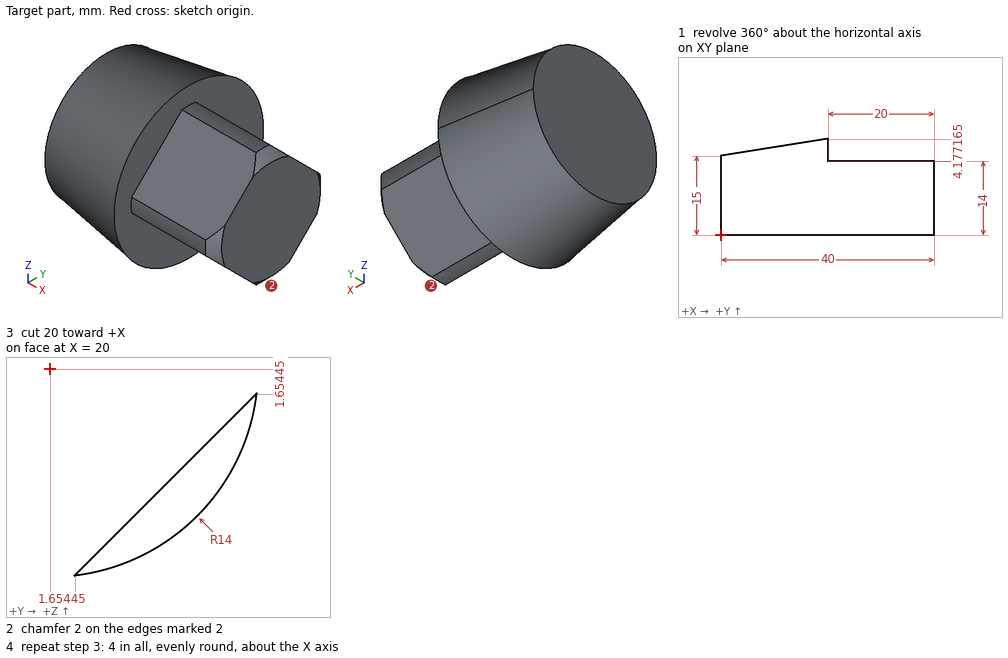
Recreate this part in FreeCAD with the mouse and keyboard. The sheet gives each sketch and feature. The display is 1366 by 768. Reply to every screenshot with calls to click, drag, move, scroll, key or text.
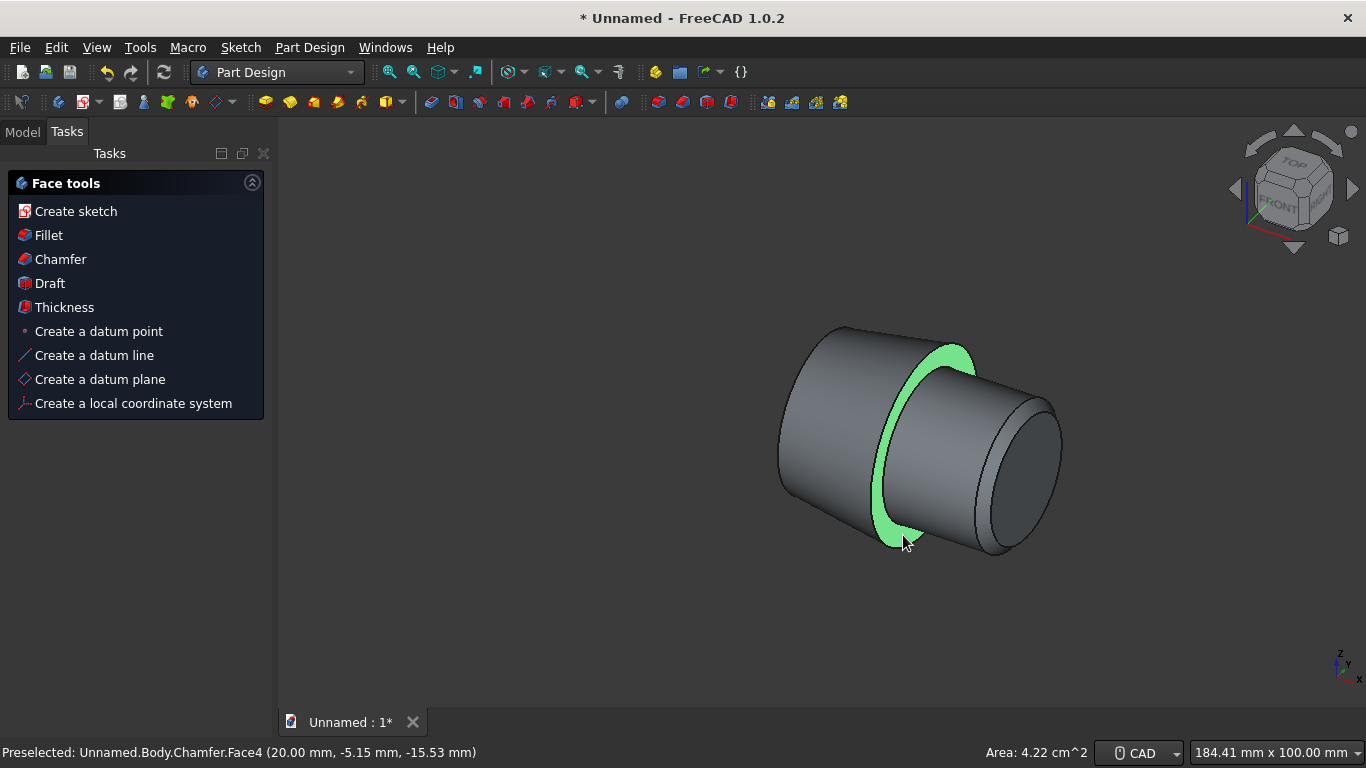
click(84, 102)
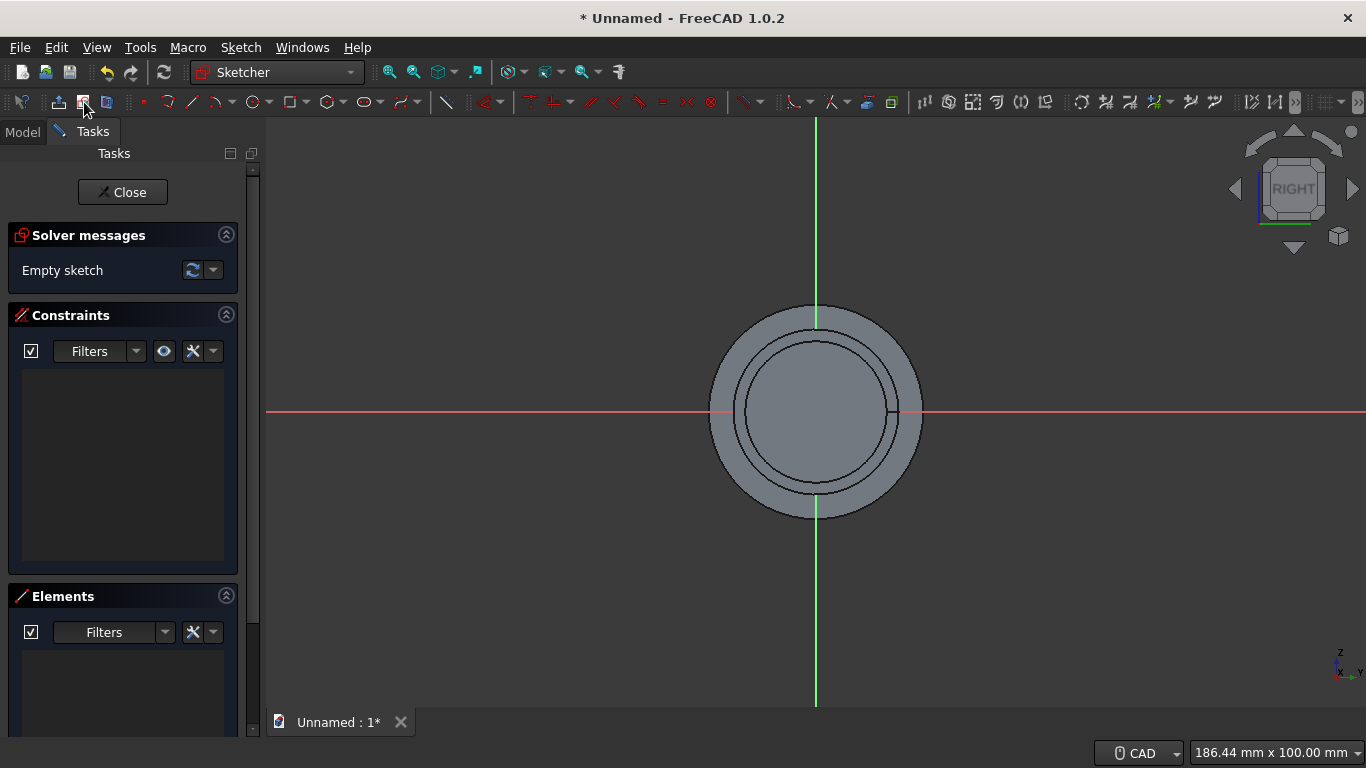
click(108, 102)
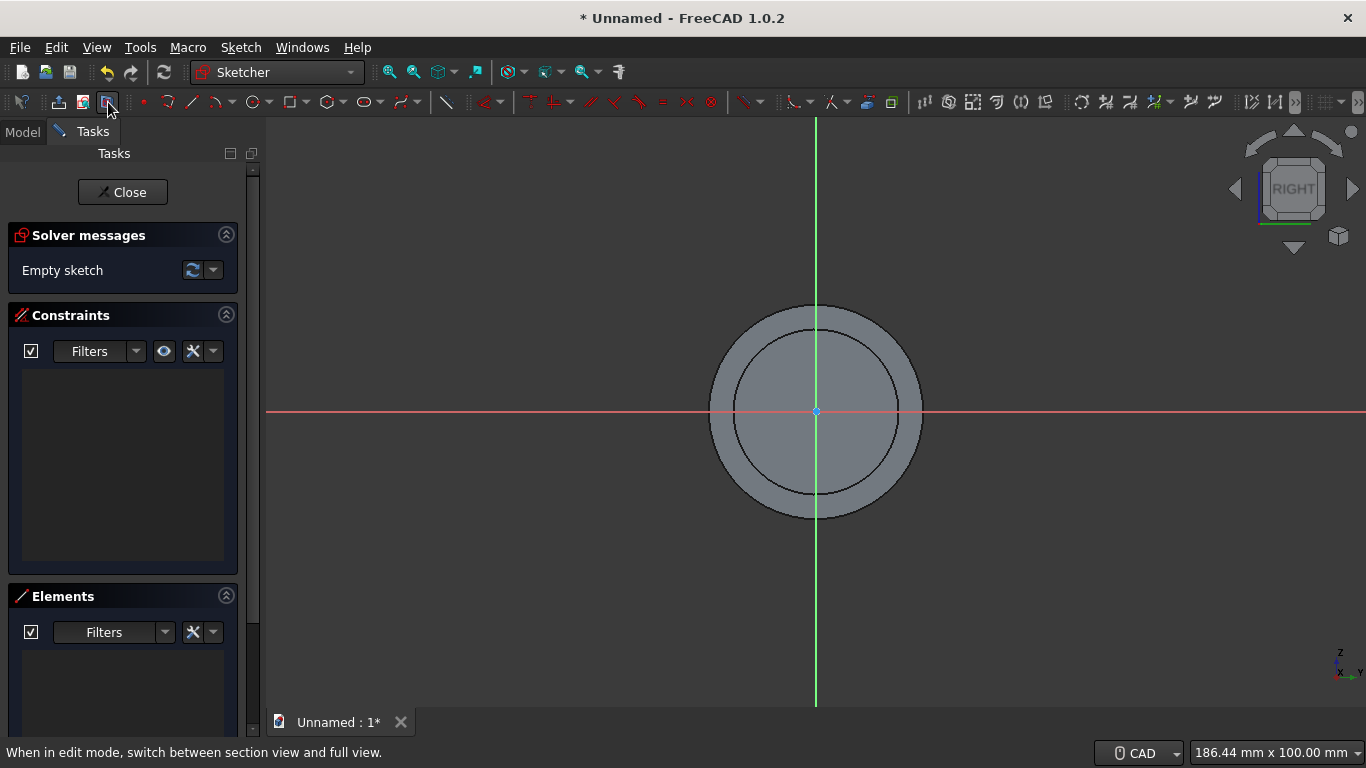
scroll(885, 463, up, 8)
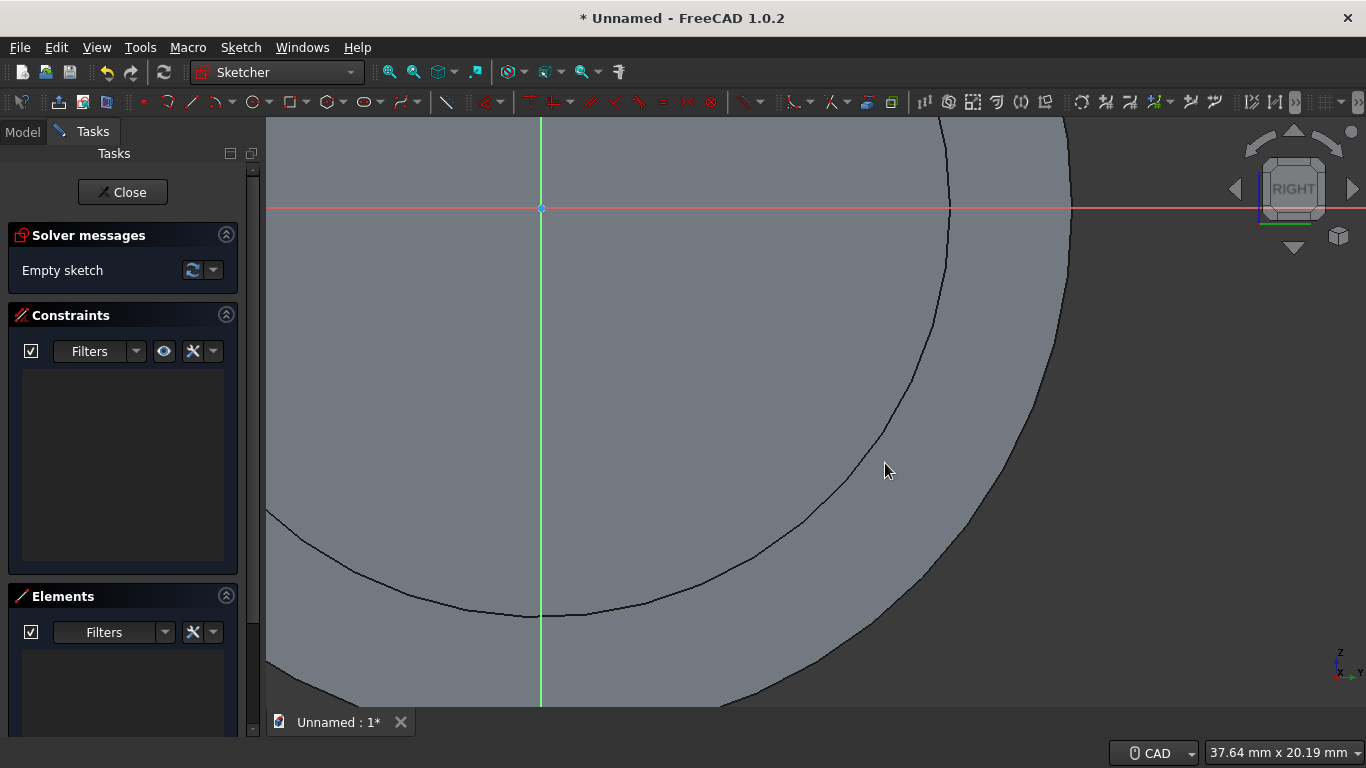
key(g)
key(l)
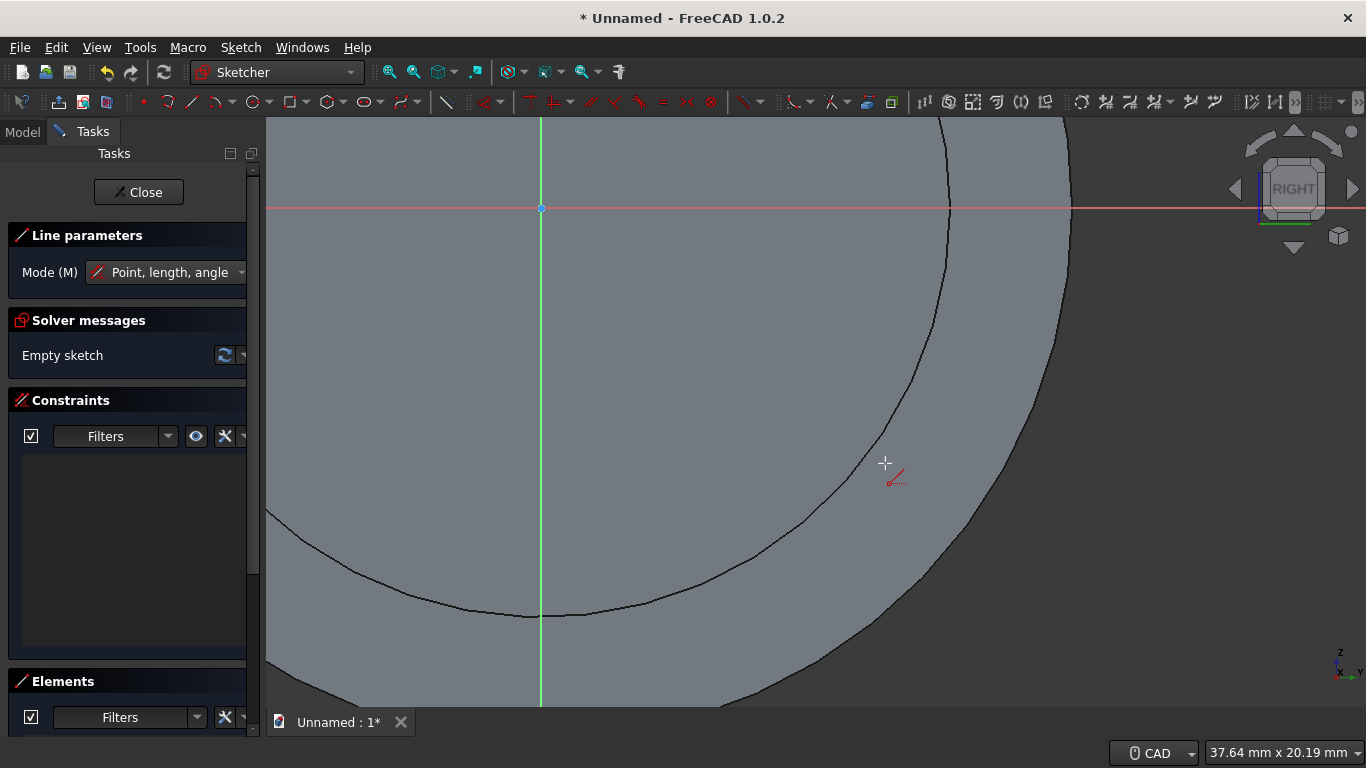
click(947, 256)
click(589, 614)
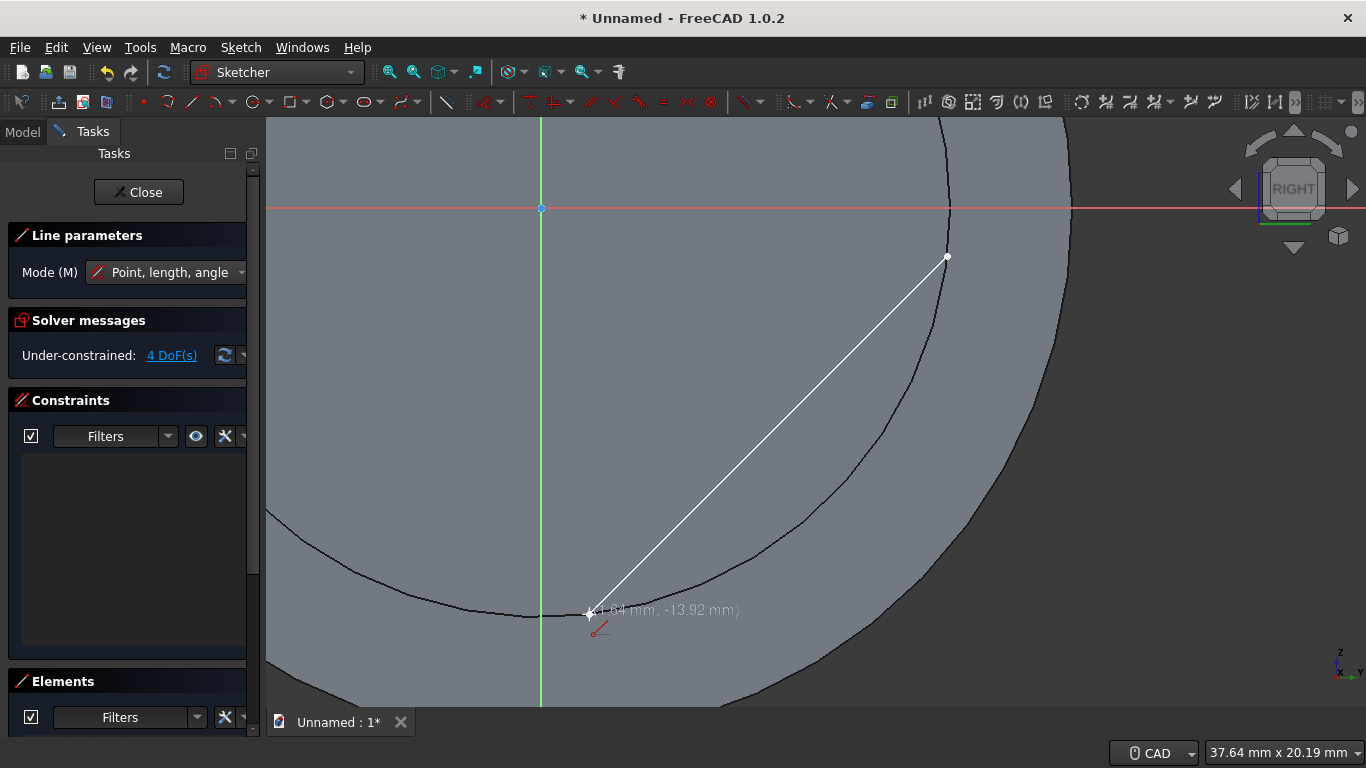
key(g)
key(3)
key(a)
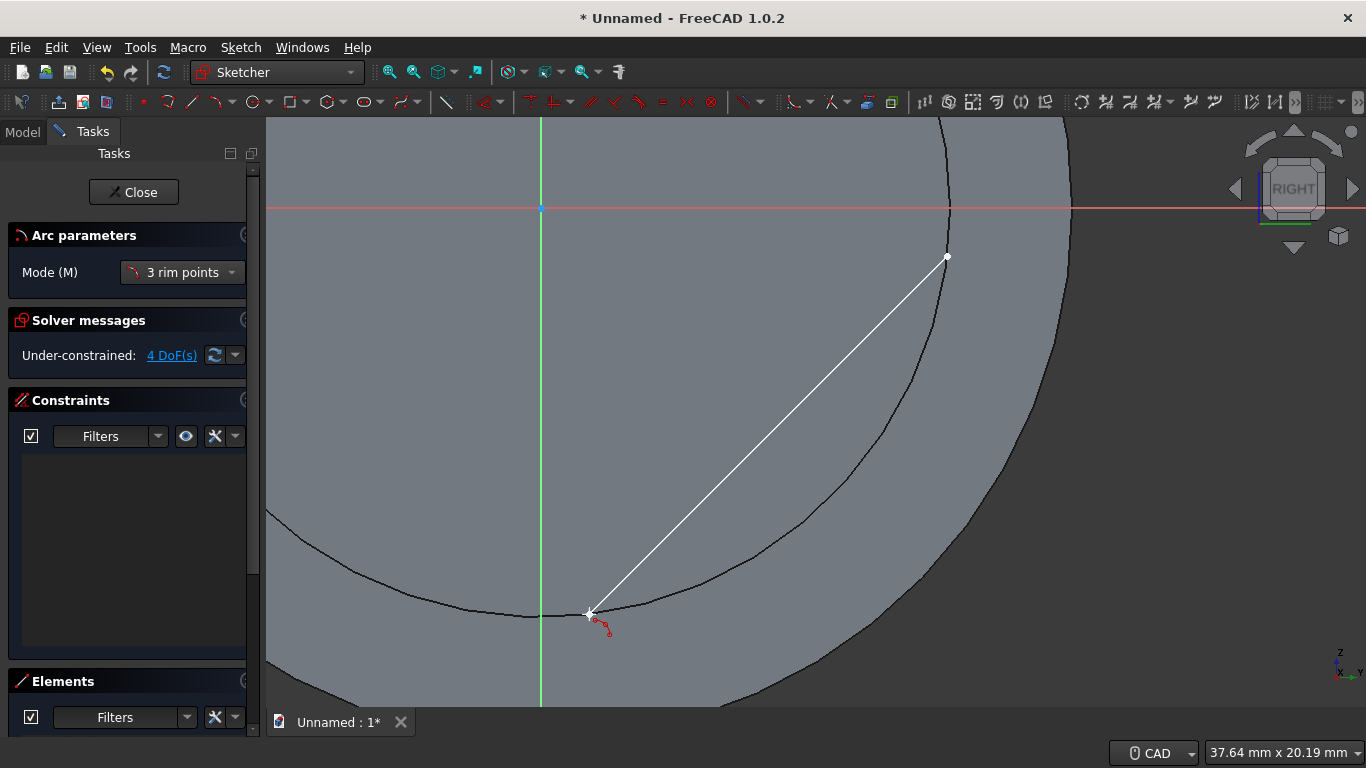
click(589, 615)
click(947, 257)
click(830, 497)
key(Escape)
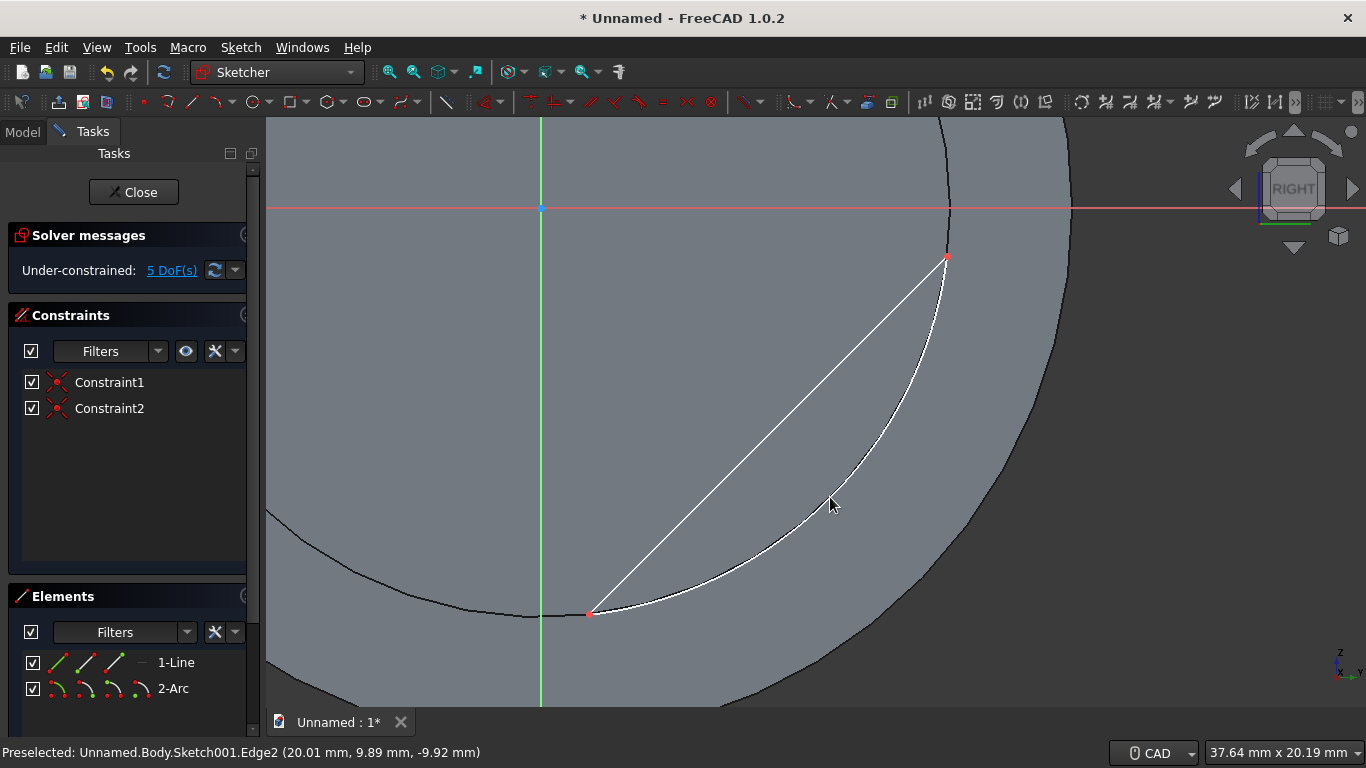
drag(531, 198, 551, 219)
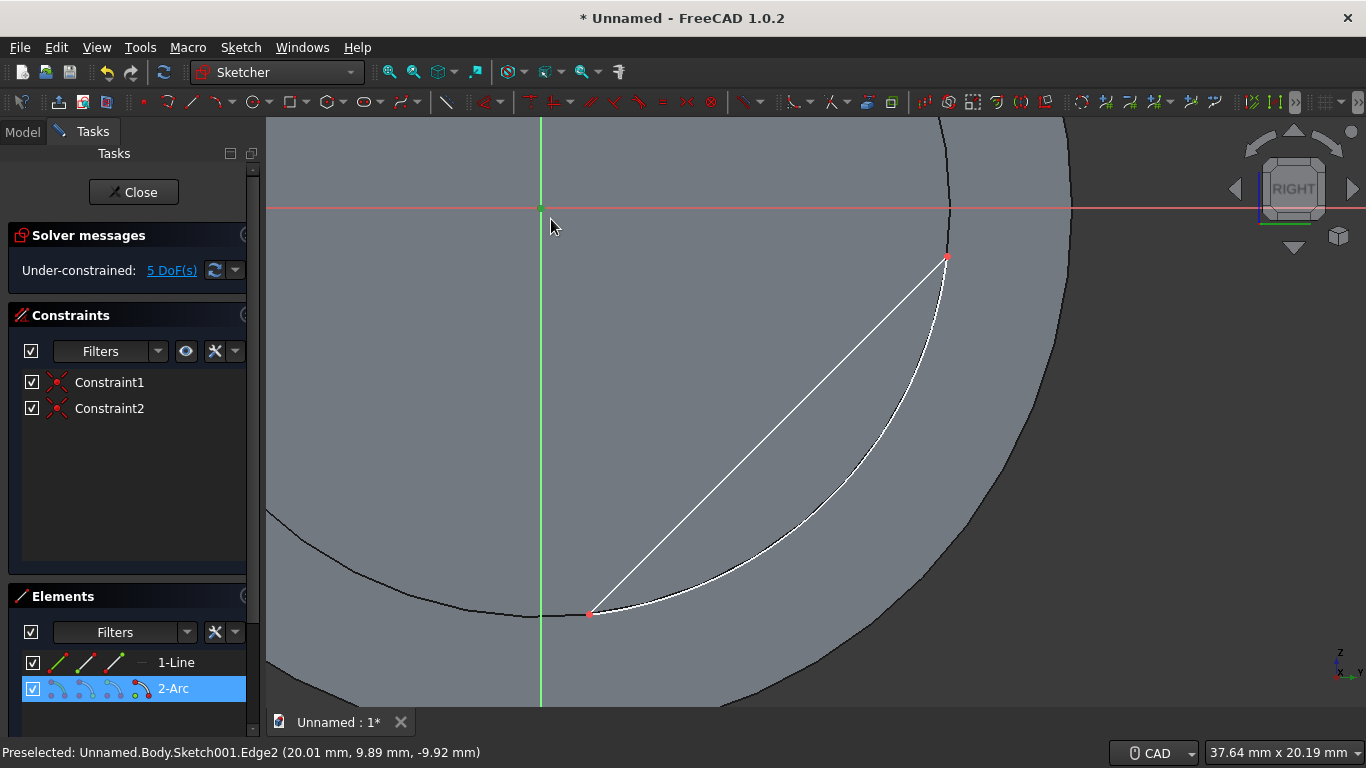
click(530, 102)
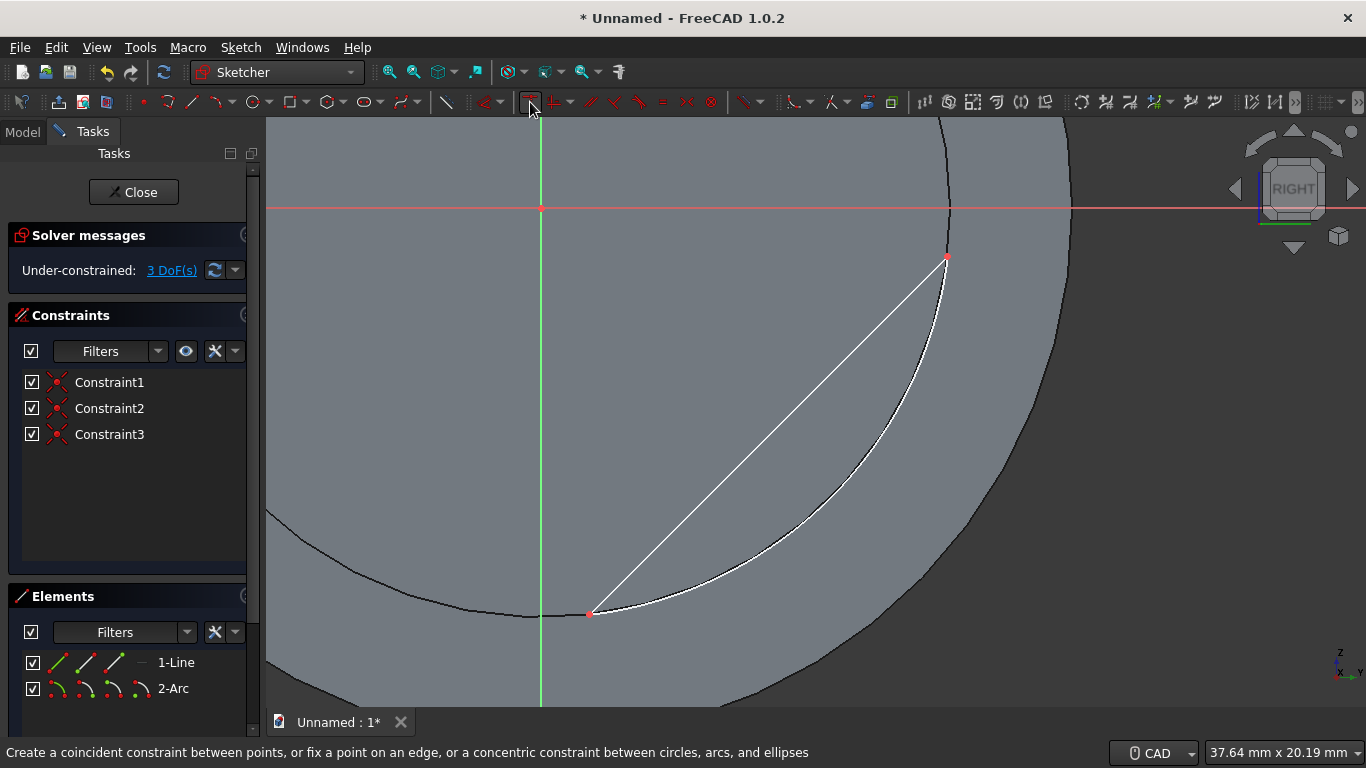
key(d)